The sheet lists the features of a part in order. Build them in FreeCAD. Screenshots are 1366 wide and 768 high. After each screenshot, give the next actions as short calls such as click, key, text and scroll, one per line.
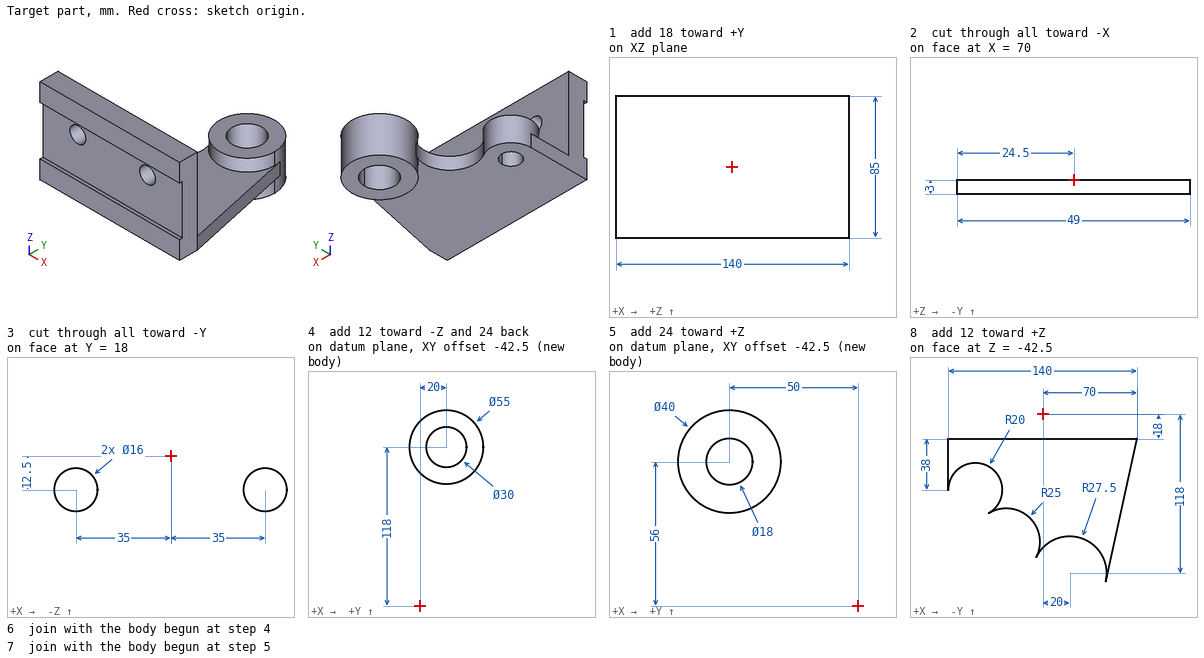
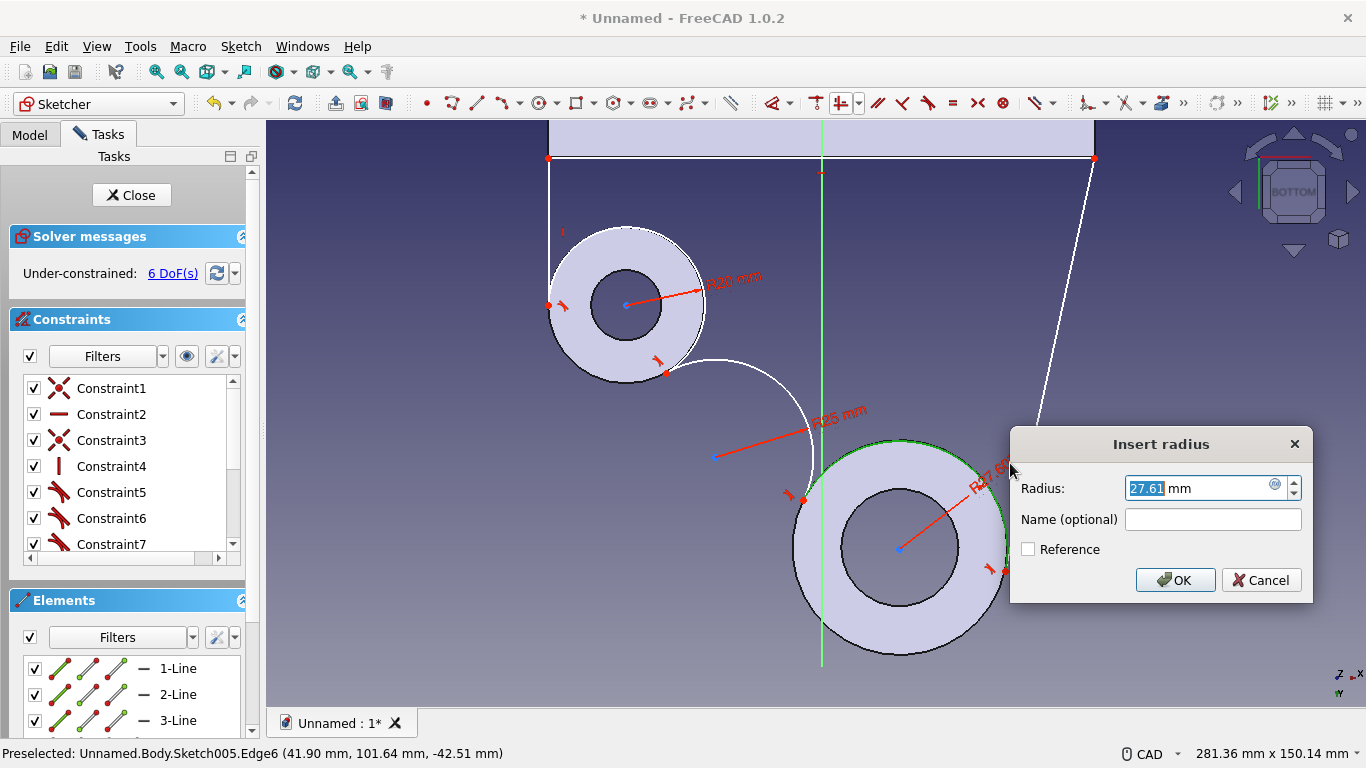
text(27.5)
key(Return)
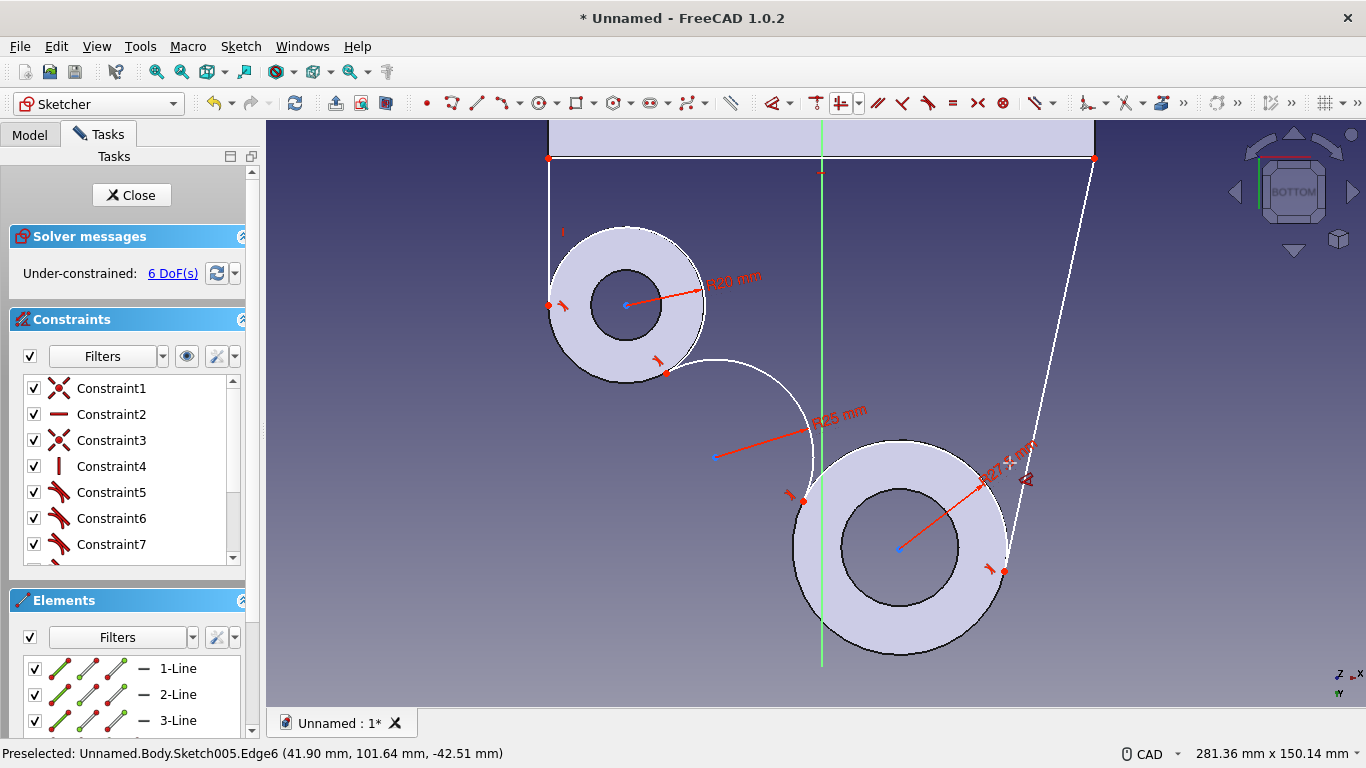
click(549, 202)
click(515, 232)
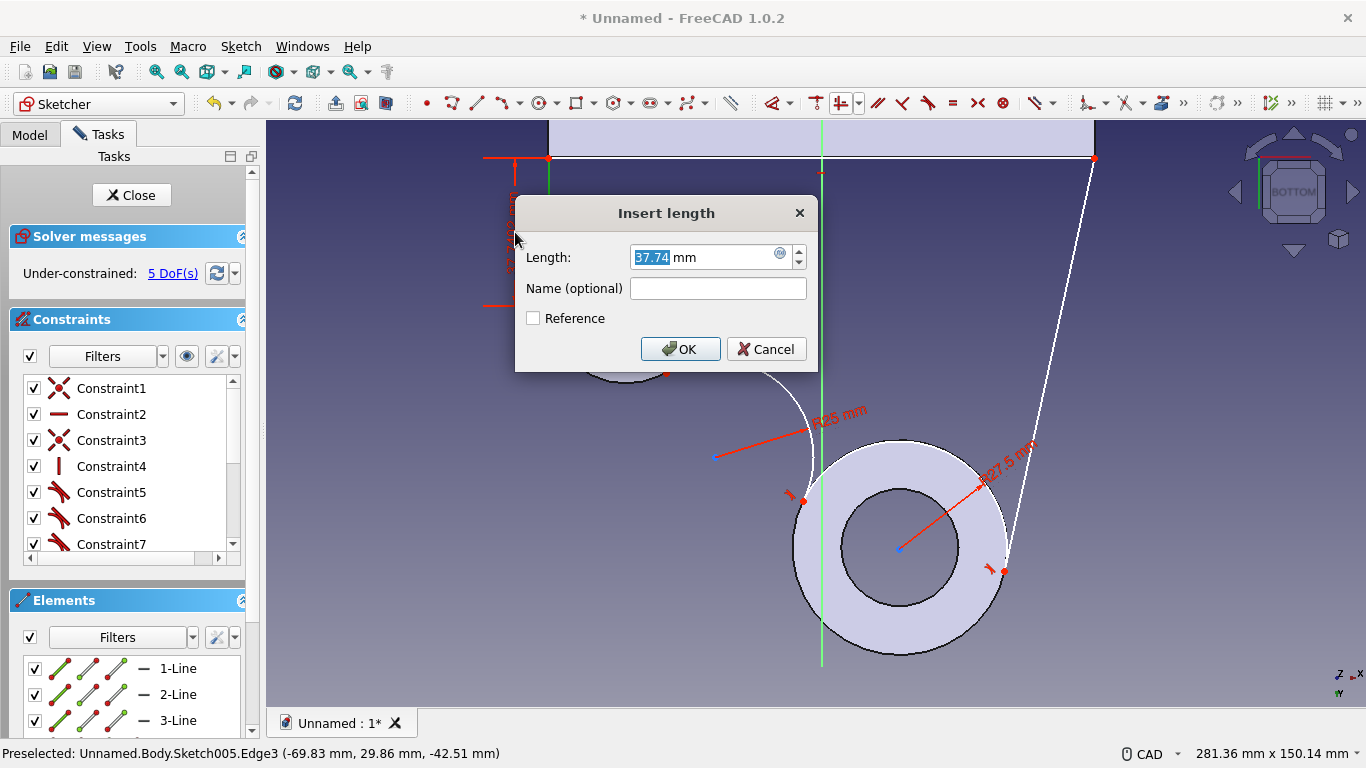
text(38)
key(Return)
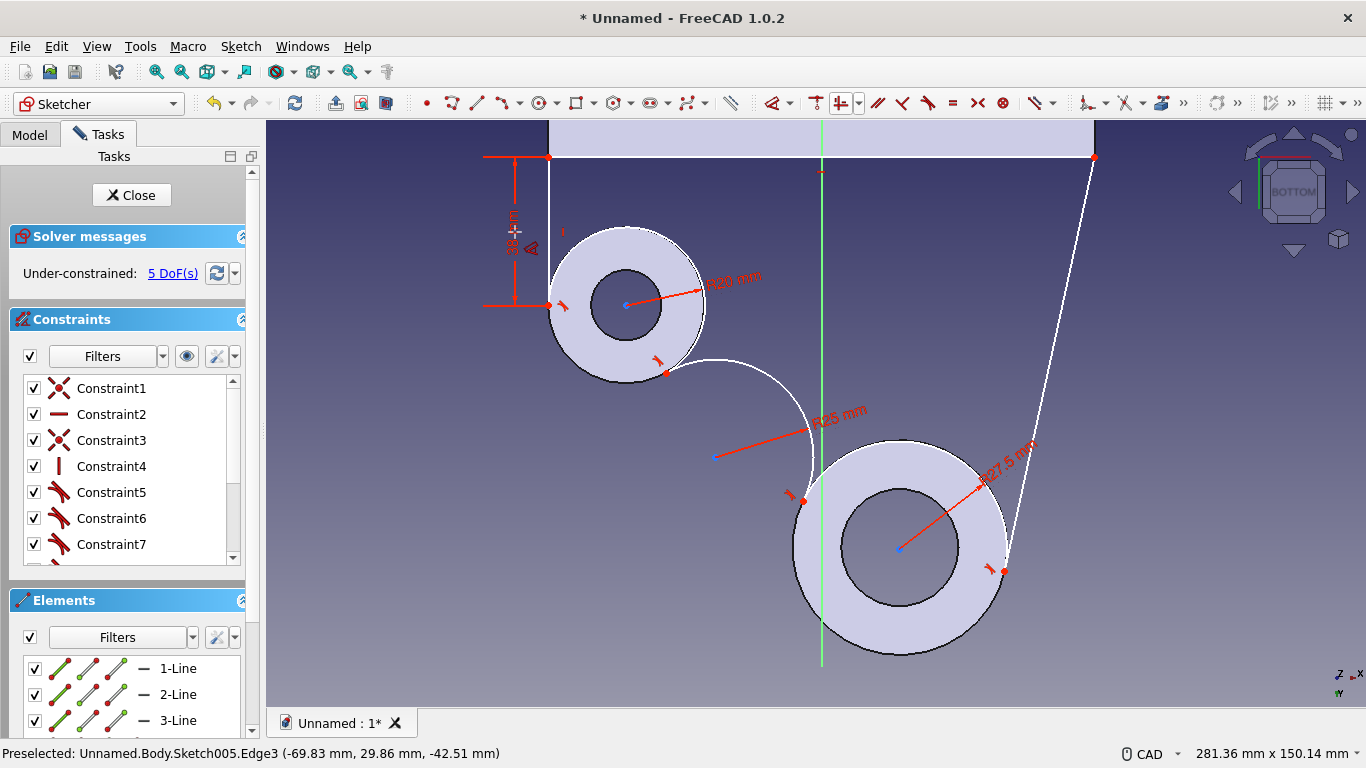
click(931, 157)
click(696, 191)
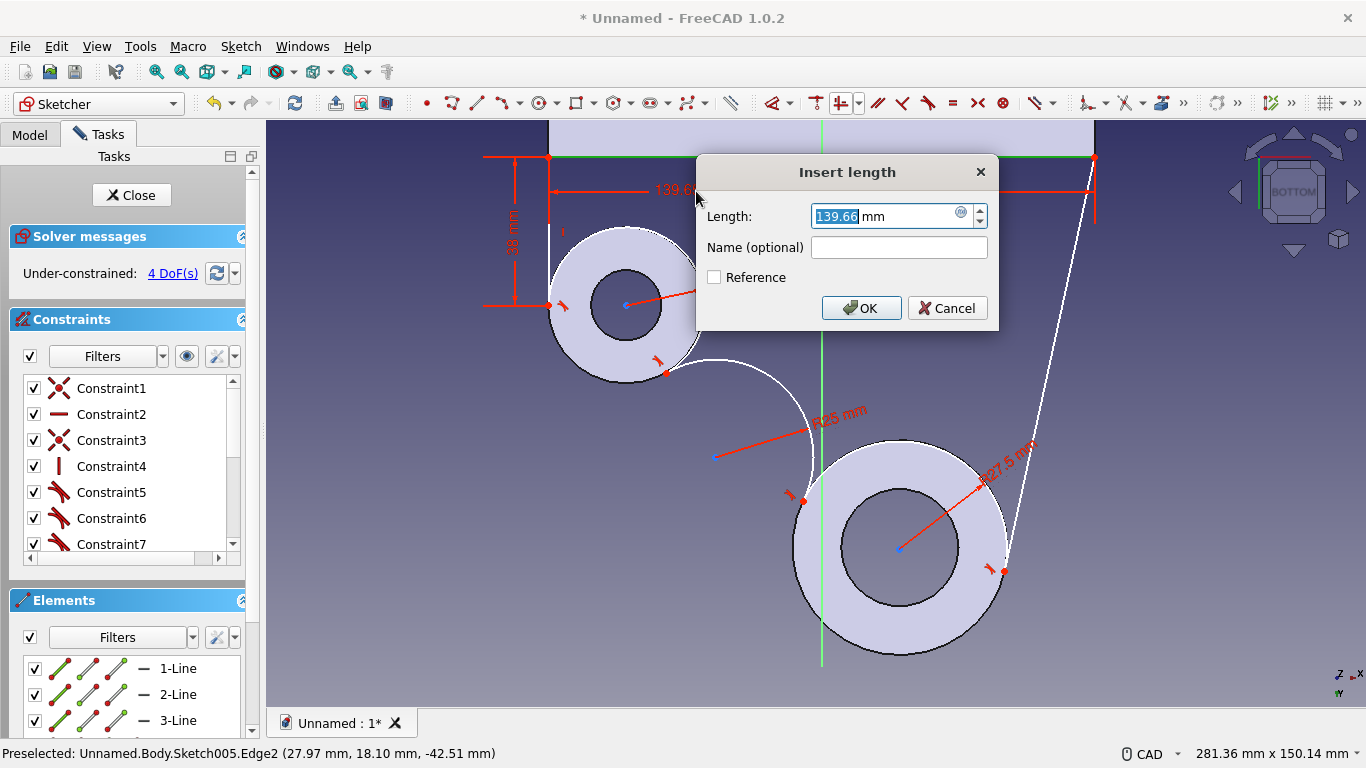
text(140)
key(Return)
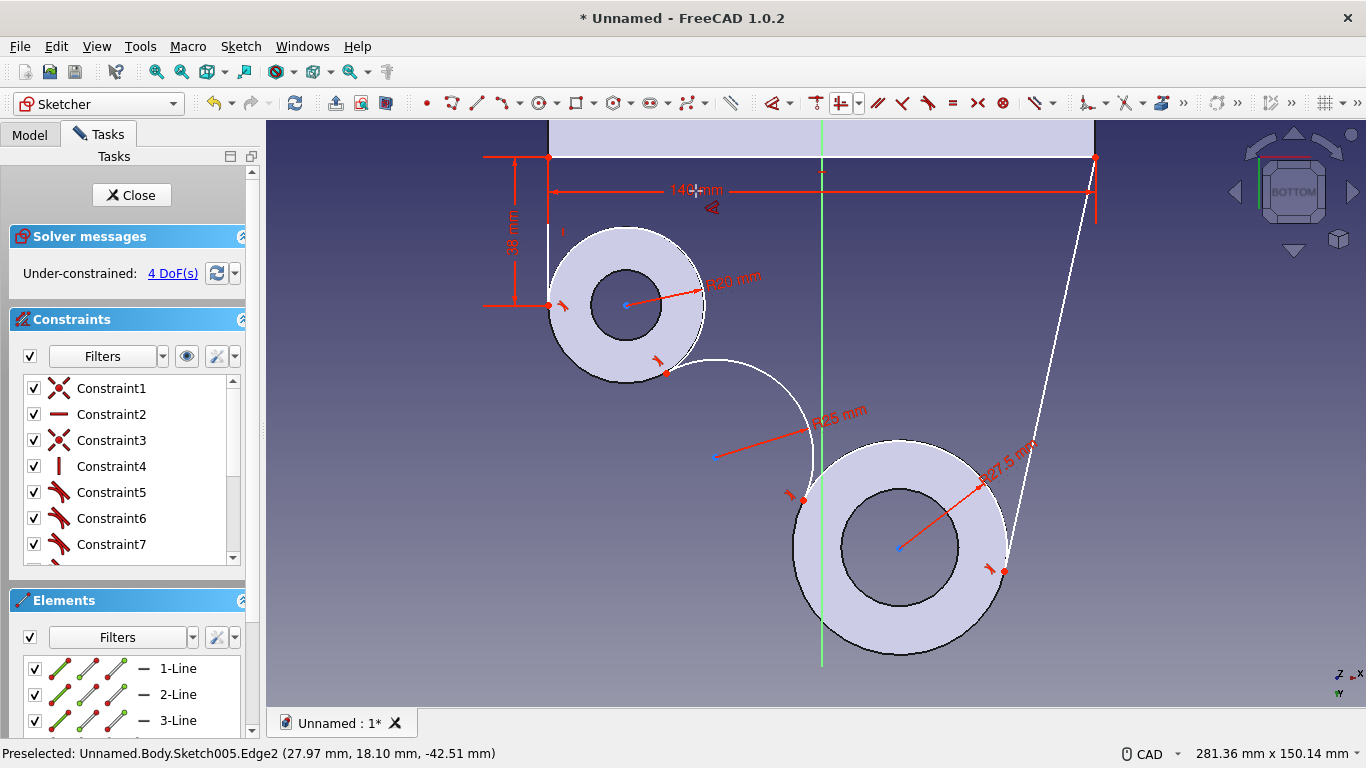
click(1096, 157)
click(959, 191)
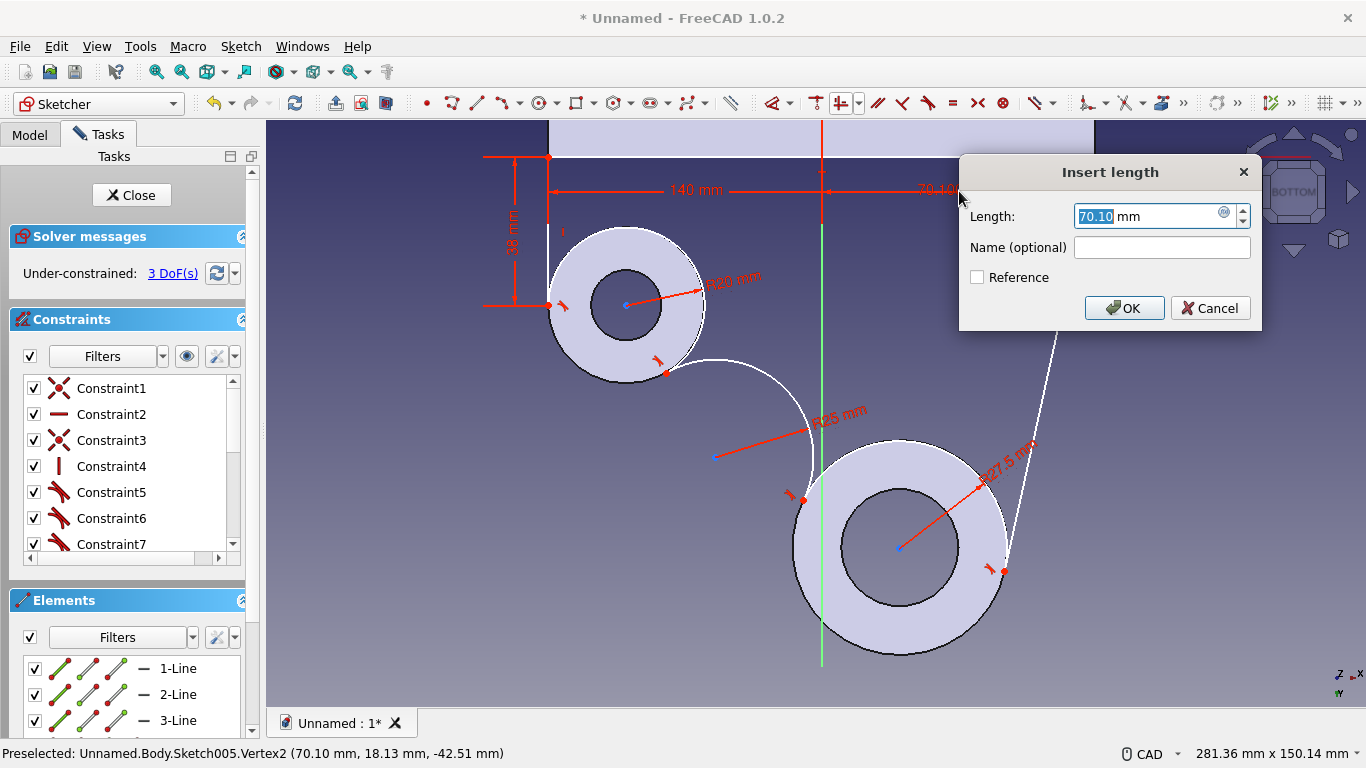
text(70)
key(Return)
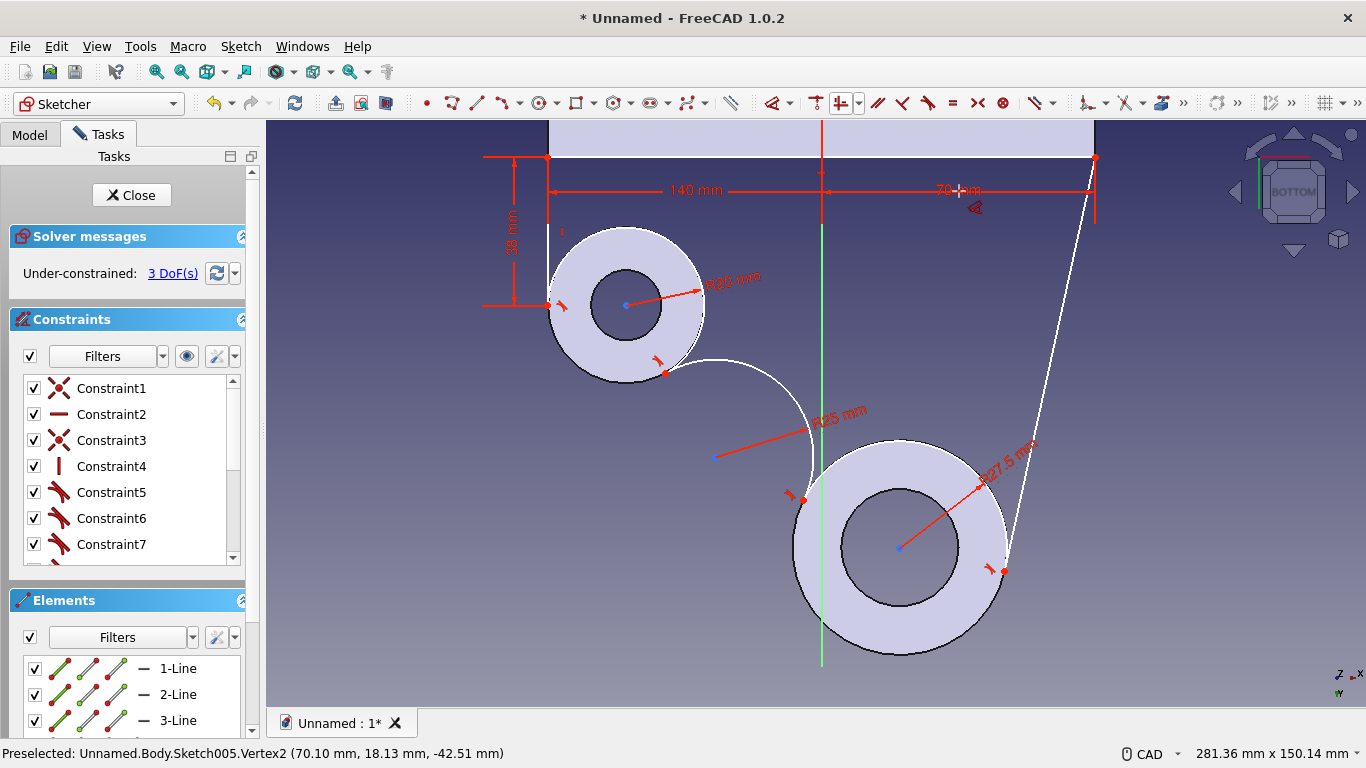
click(1095, 157)
click(1129, 153)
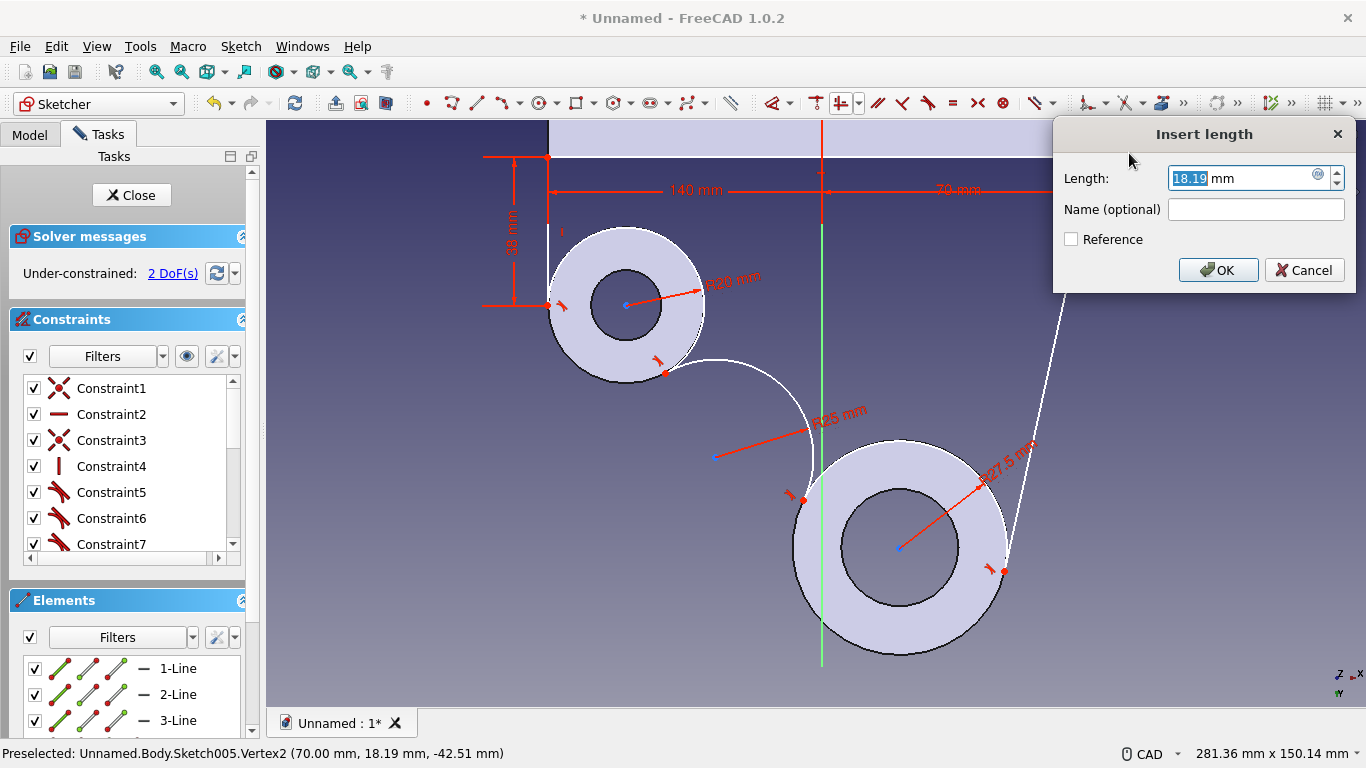
text(18)
key(Return)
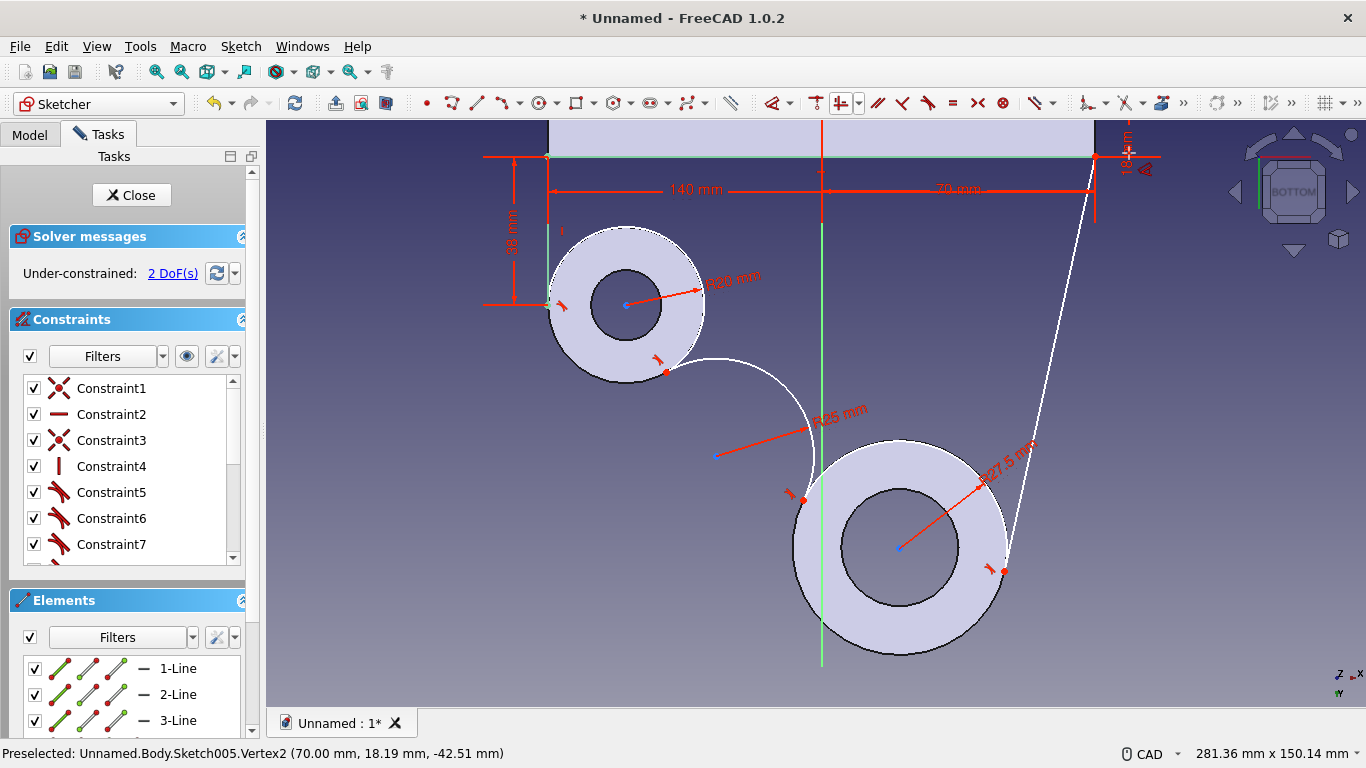
click(899, 549)
click(861, 583)